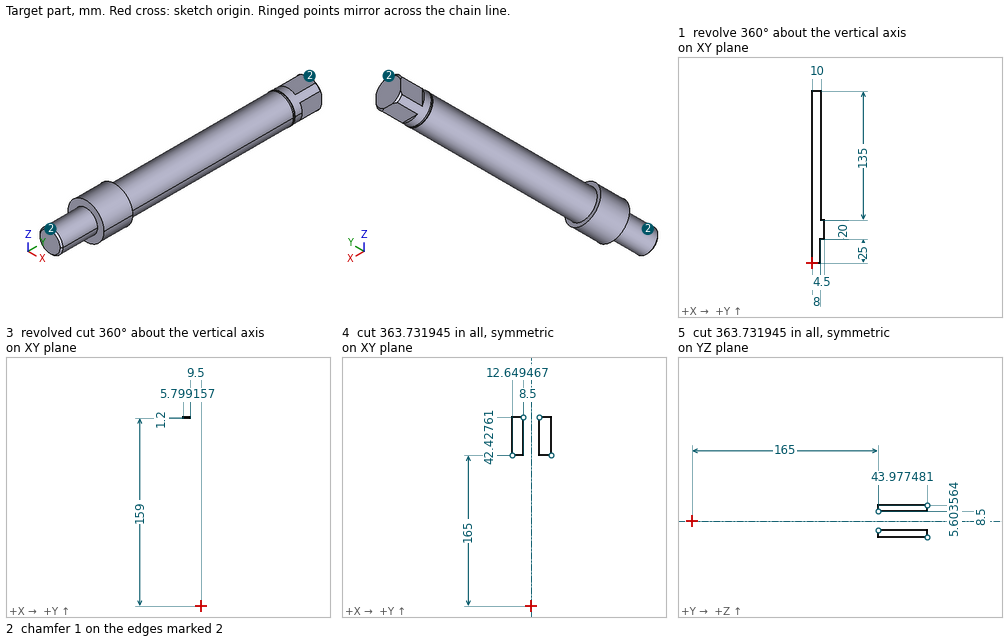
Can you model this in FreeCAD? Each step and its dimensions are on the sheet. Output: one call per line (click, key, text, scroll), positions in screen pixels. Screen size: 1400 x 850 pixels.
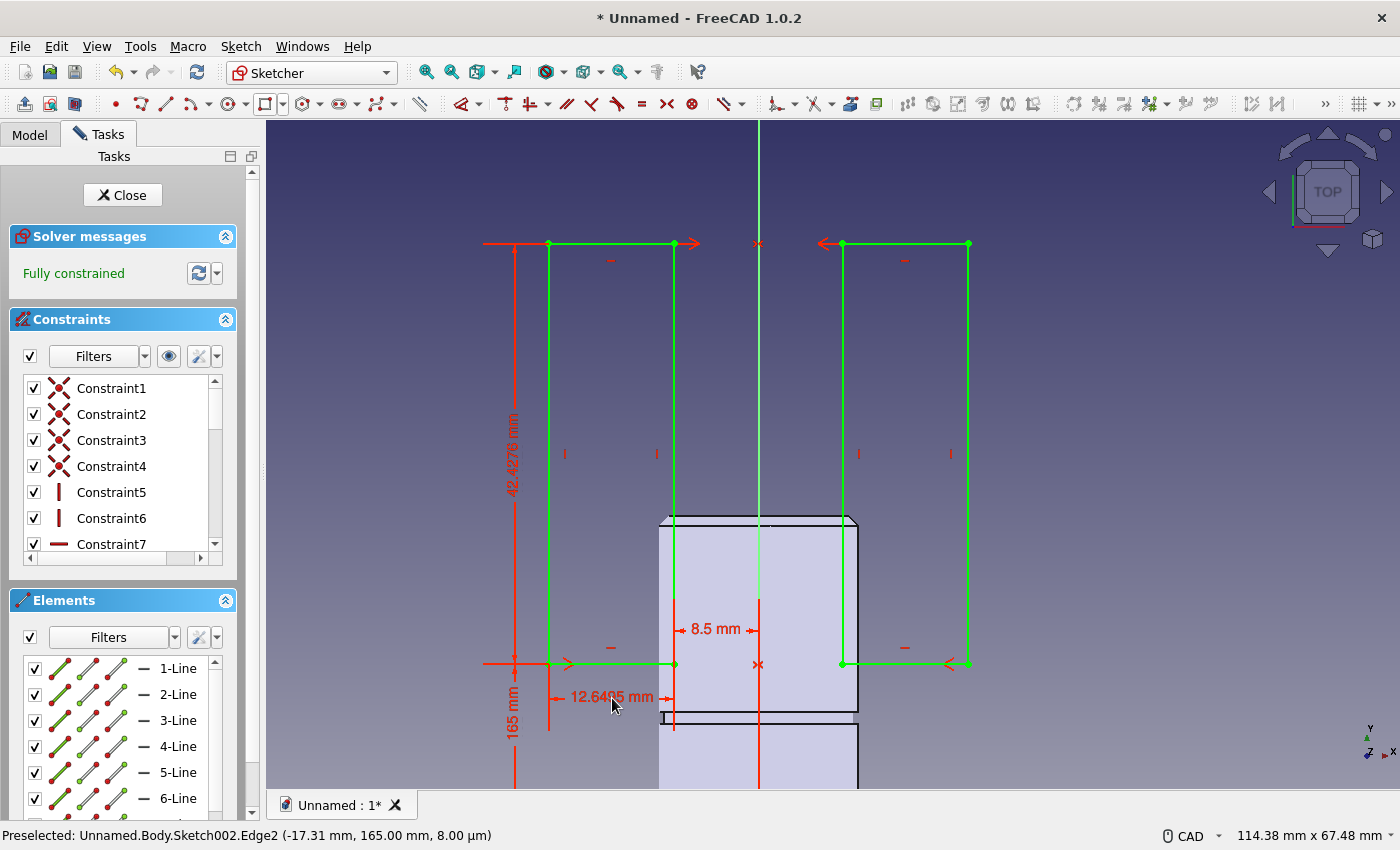
click(123, 195)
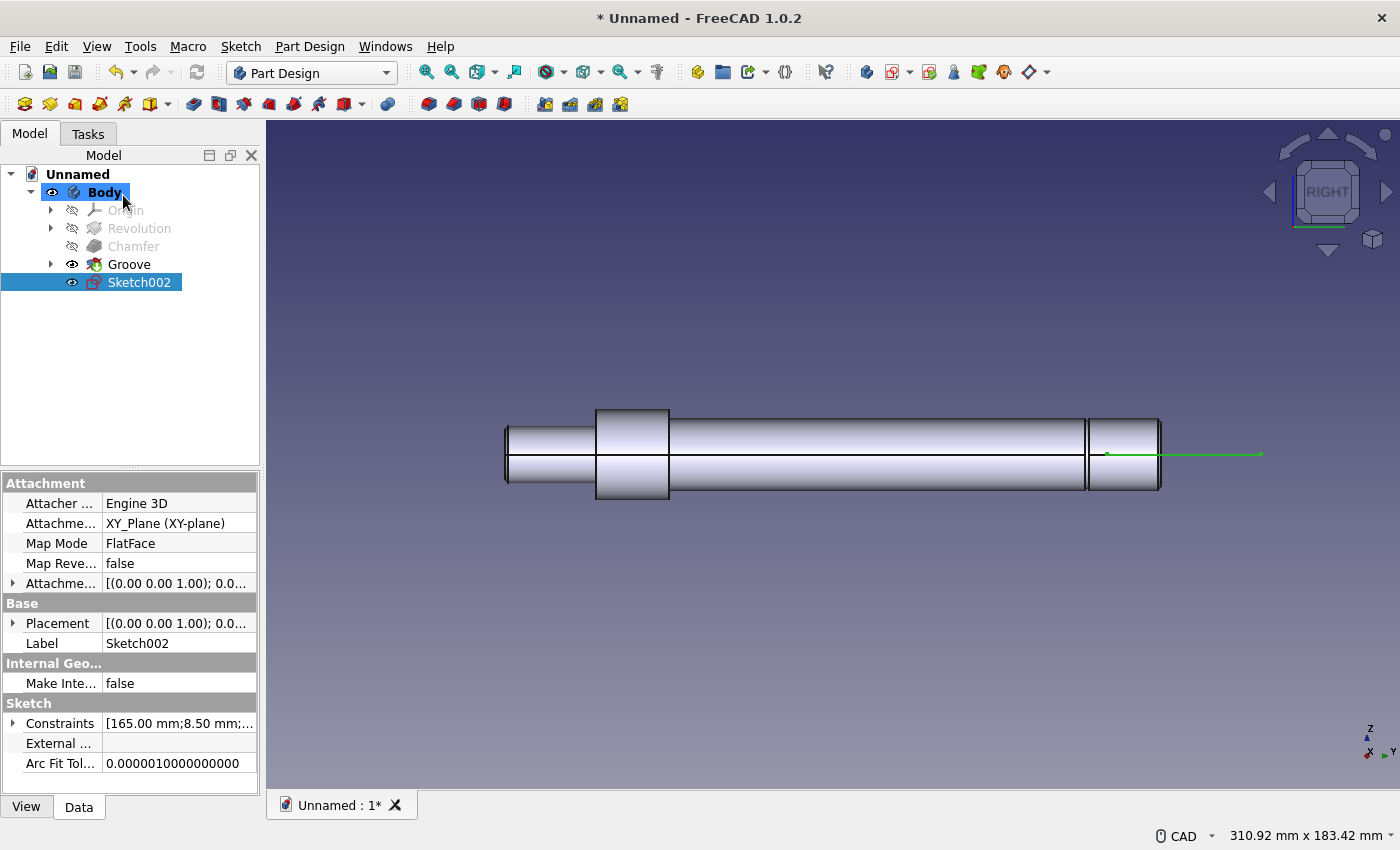
click(194, 104)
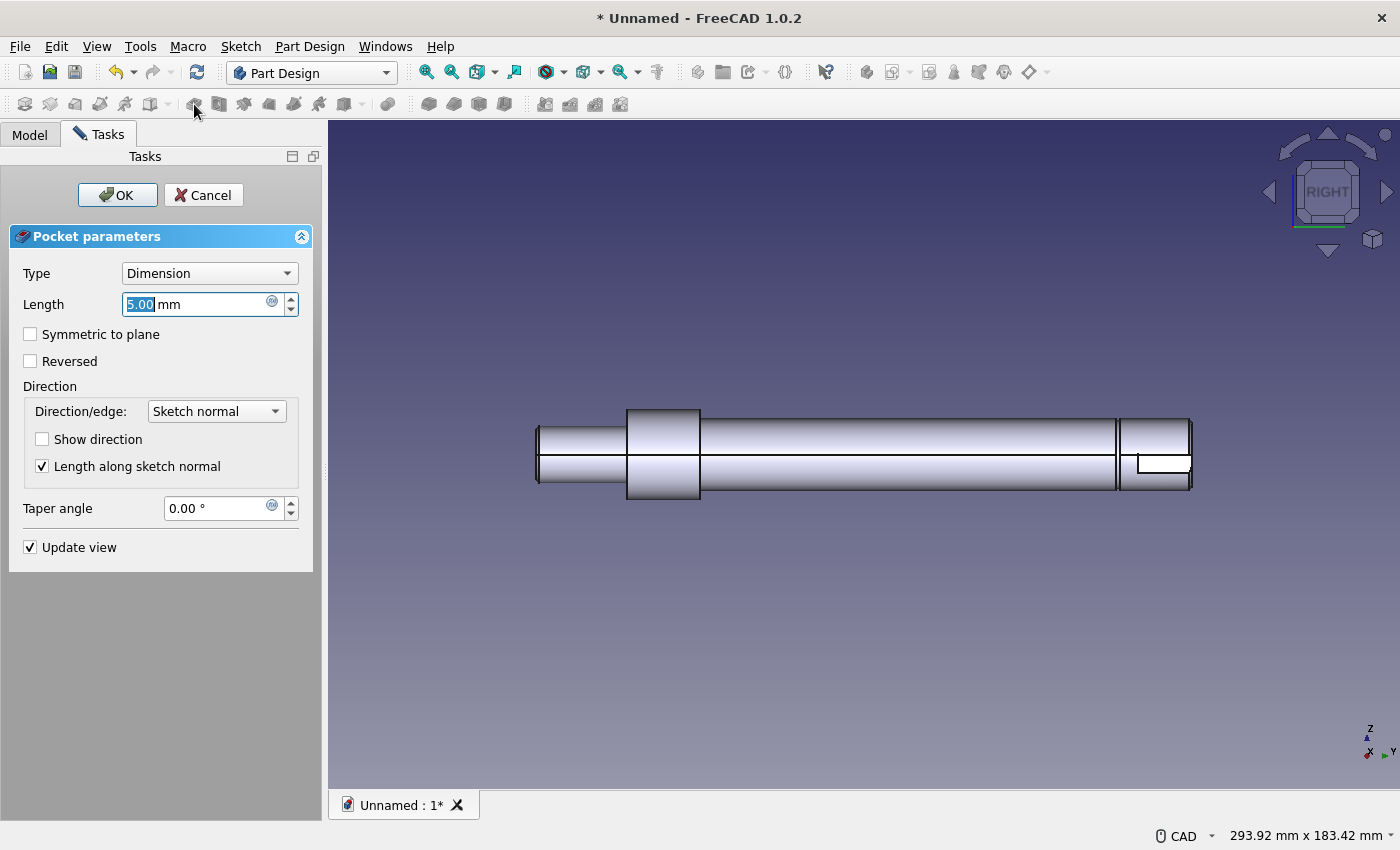
text(363.731945)
key(Tab)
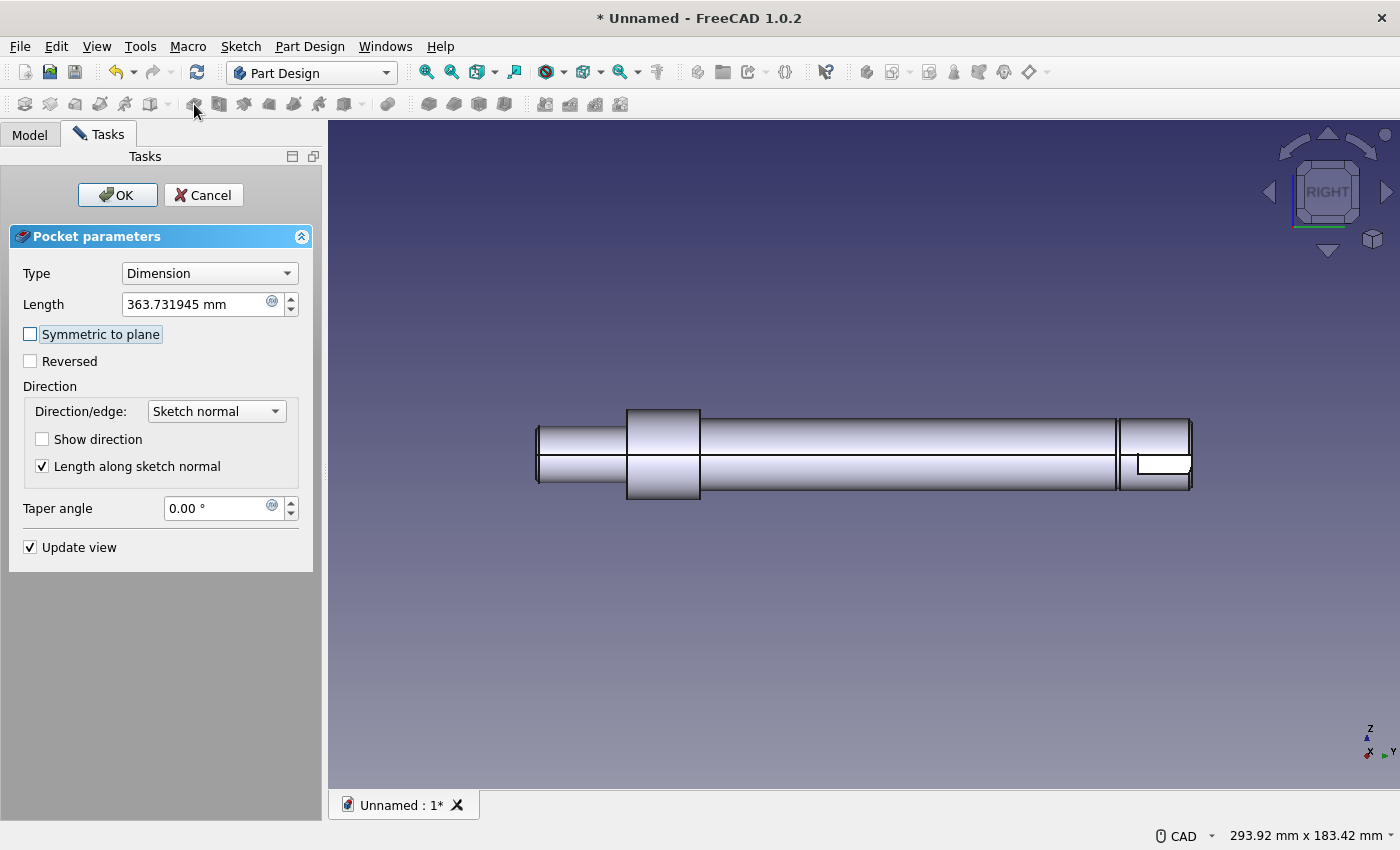
click(31, 334)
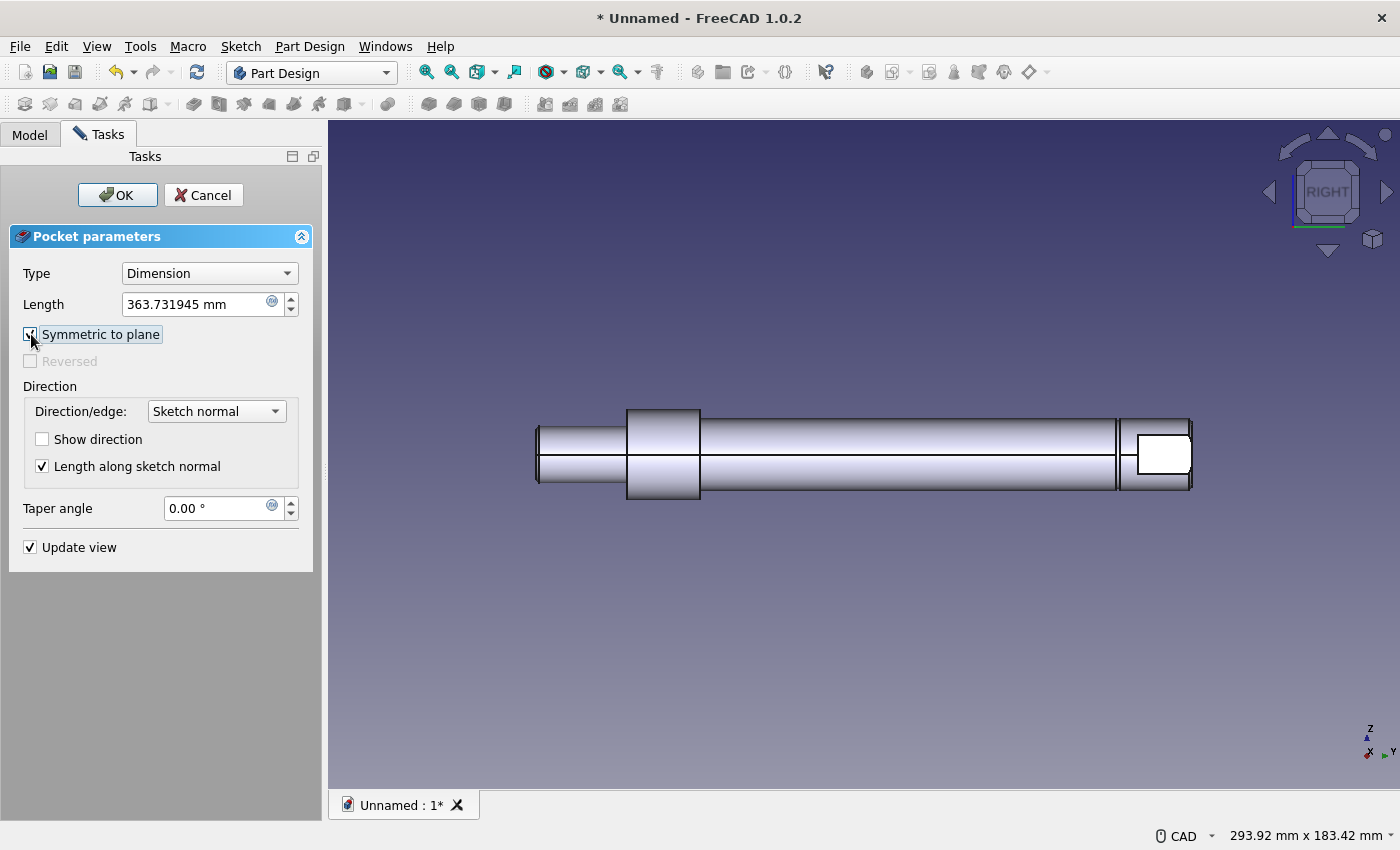
click(118, 195)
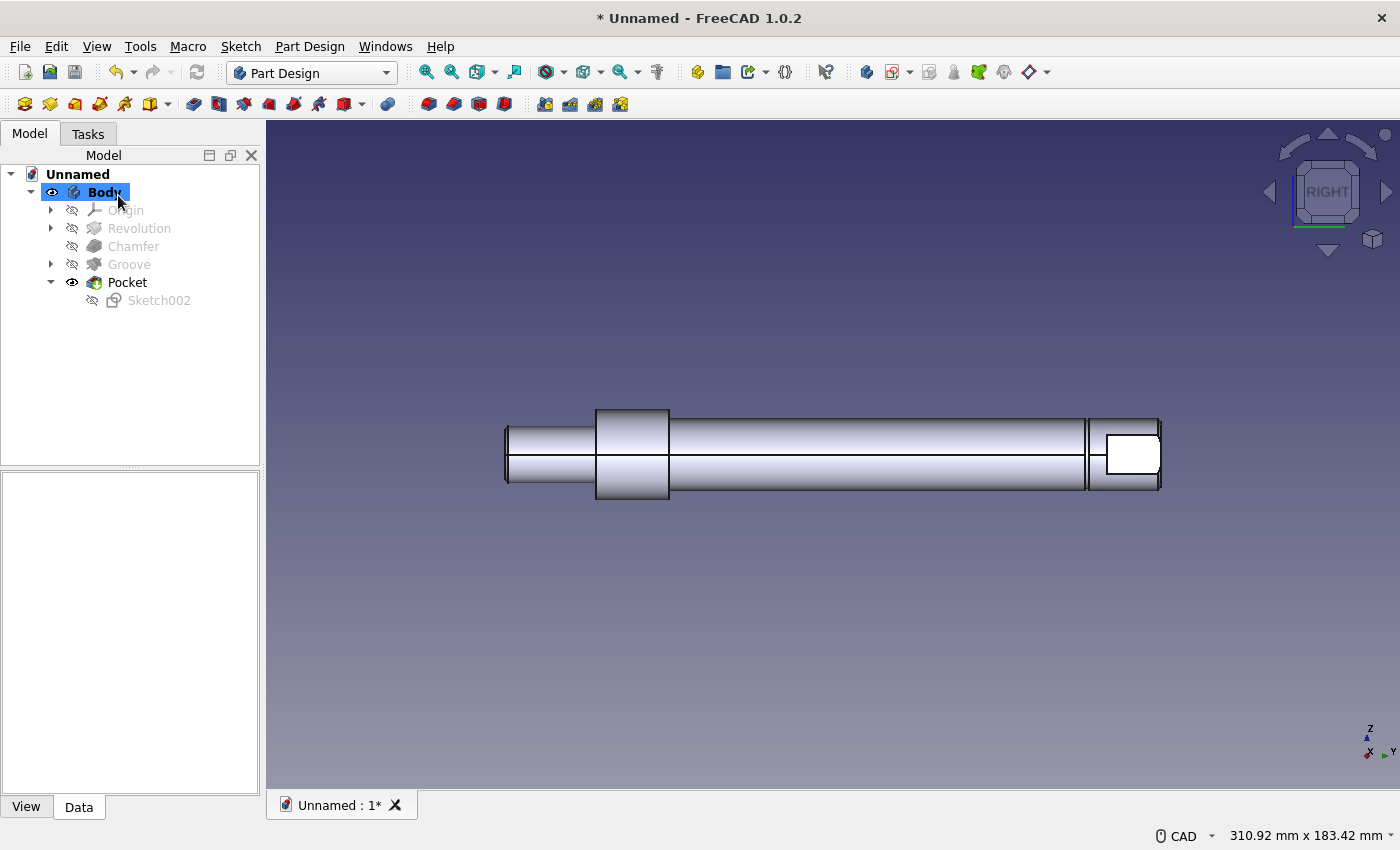
click(892, 72)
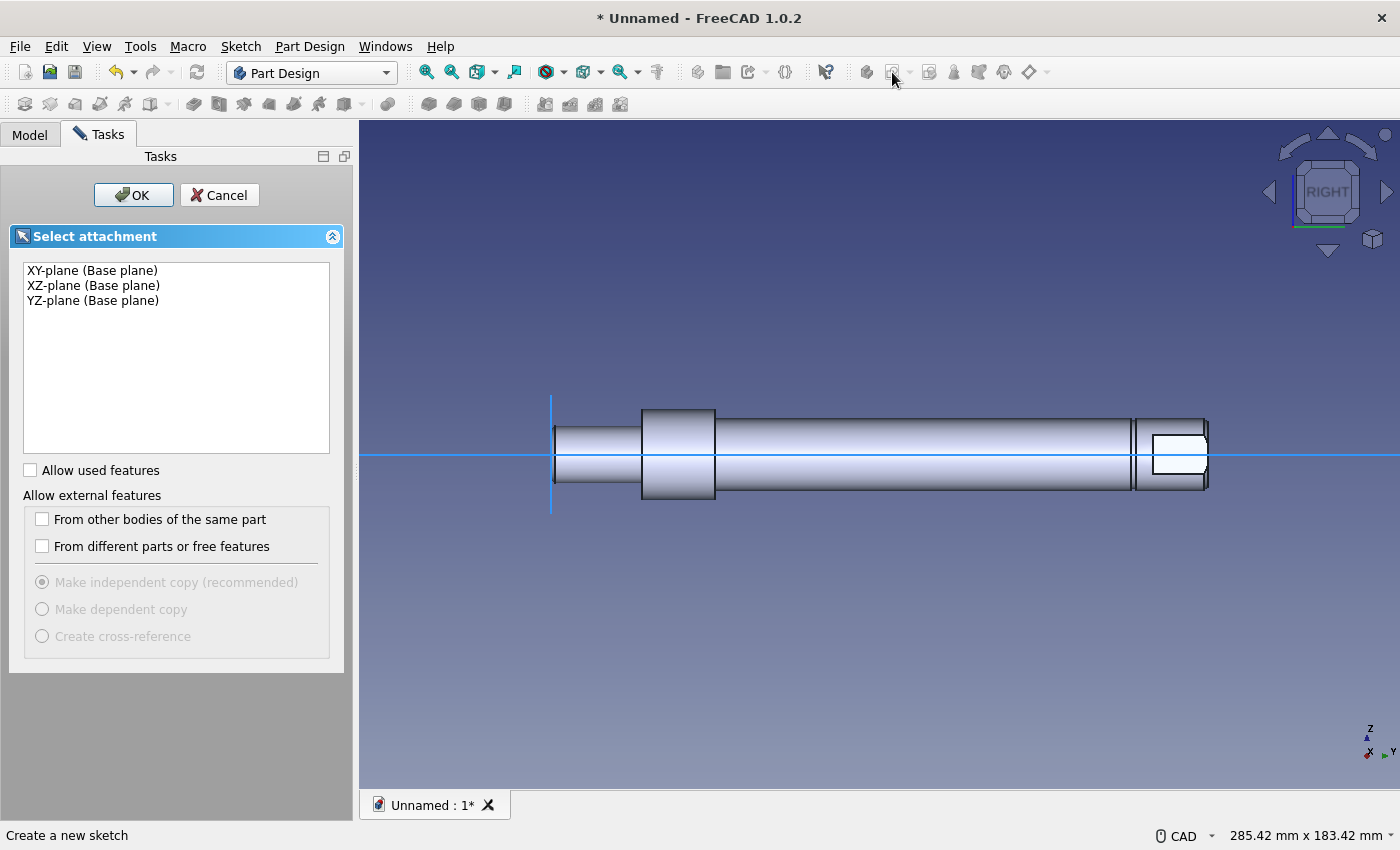
click(84, 300)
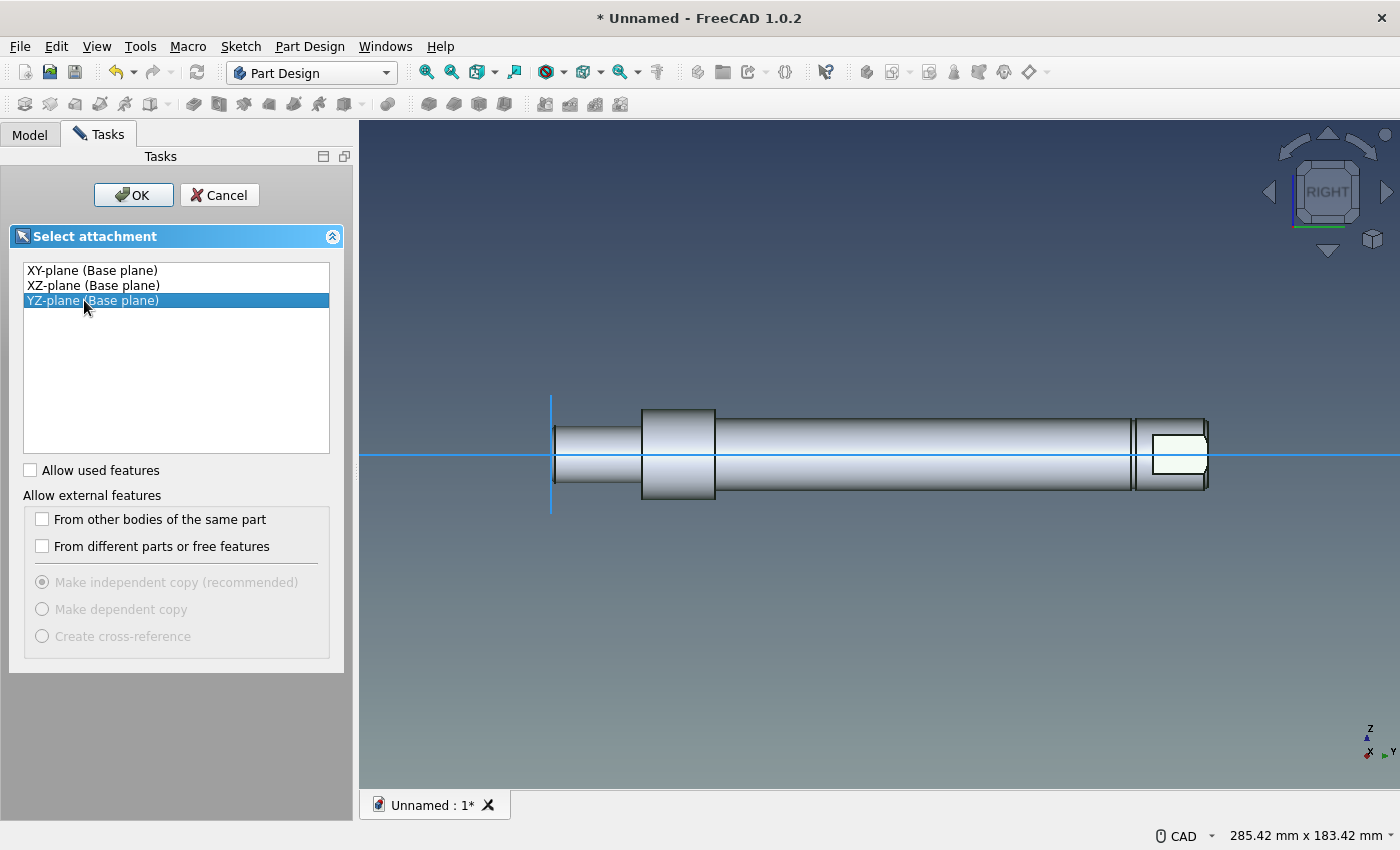
click(134, 195)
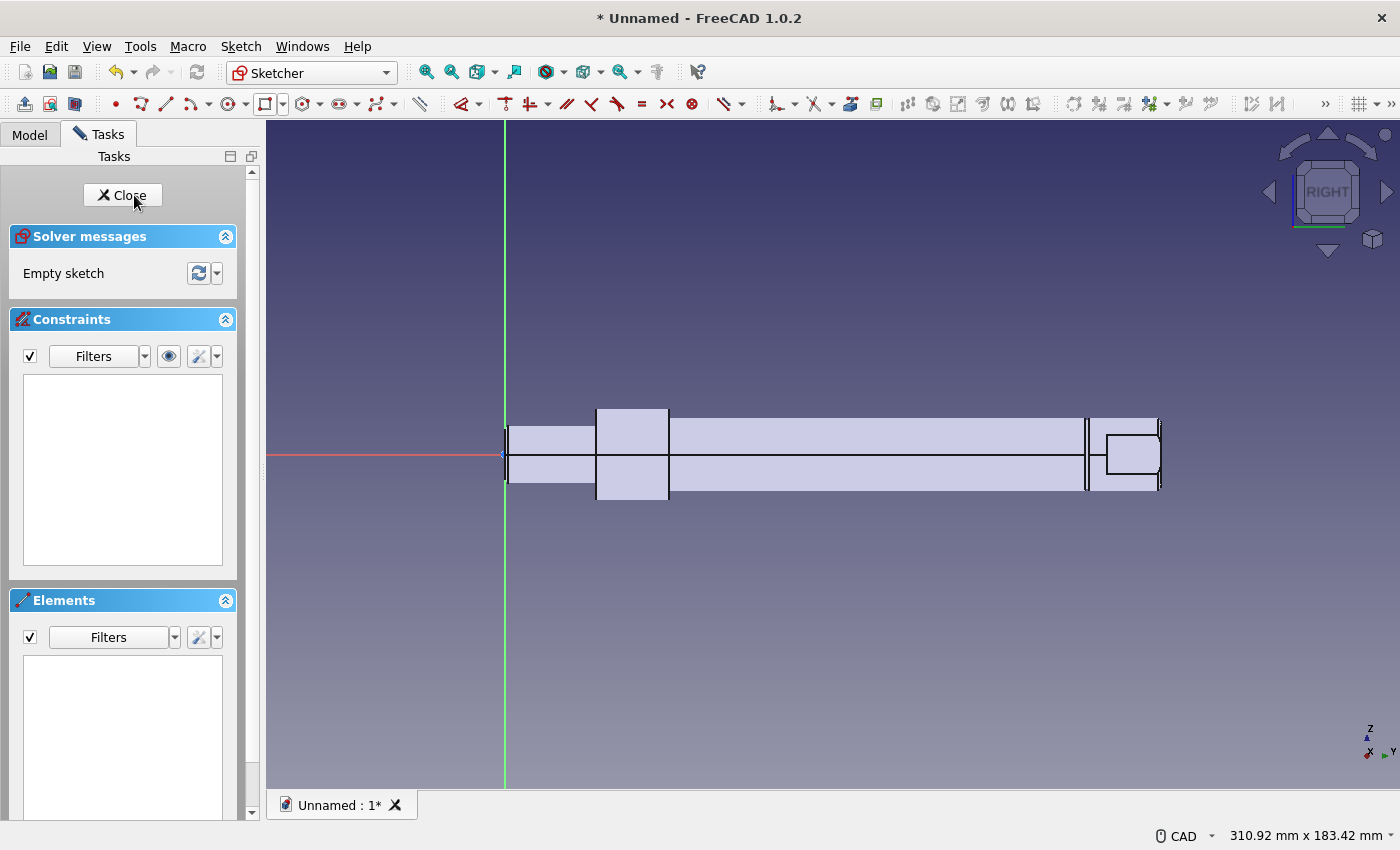
key(q)
key(s)